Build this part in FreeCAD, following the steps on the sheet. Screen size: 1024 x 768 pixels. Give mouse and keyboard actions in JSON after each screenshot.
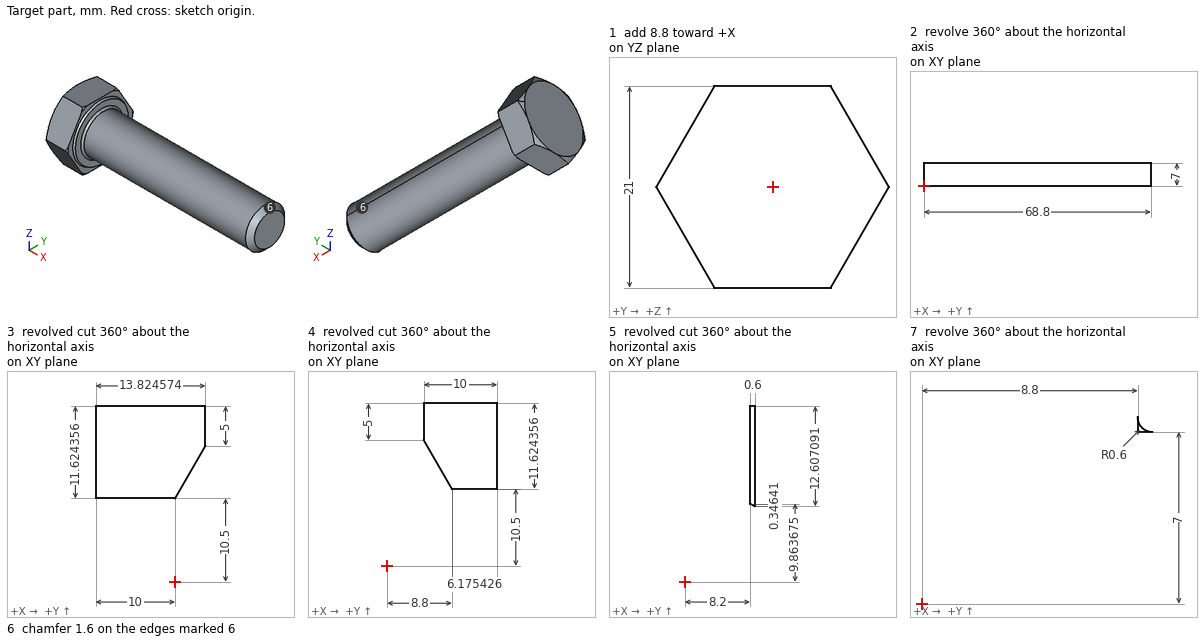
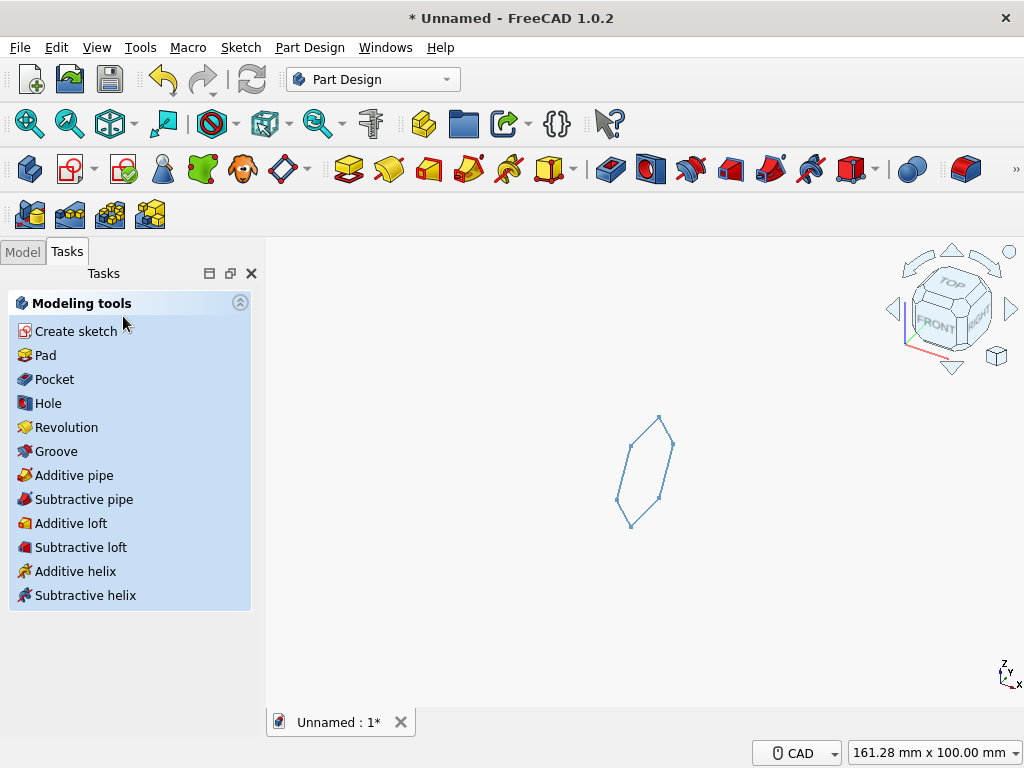
{"action": "left_click", "coordinate": [350, 170]}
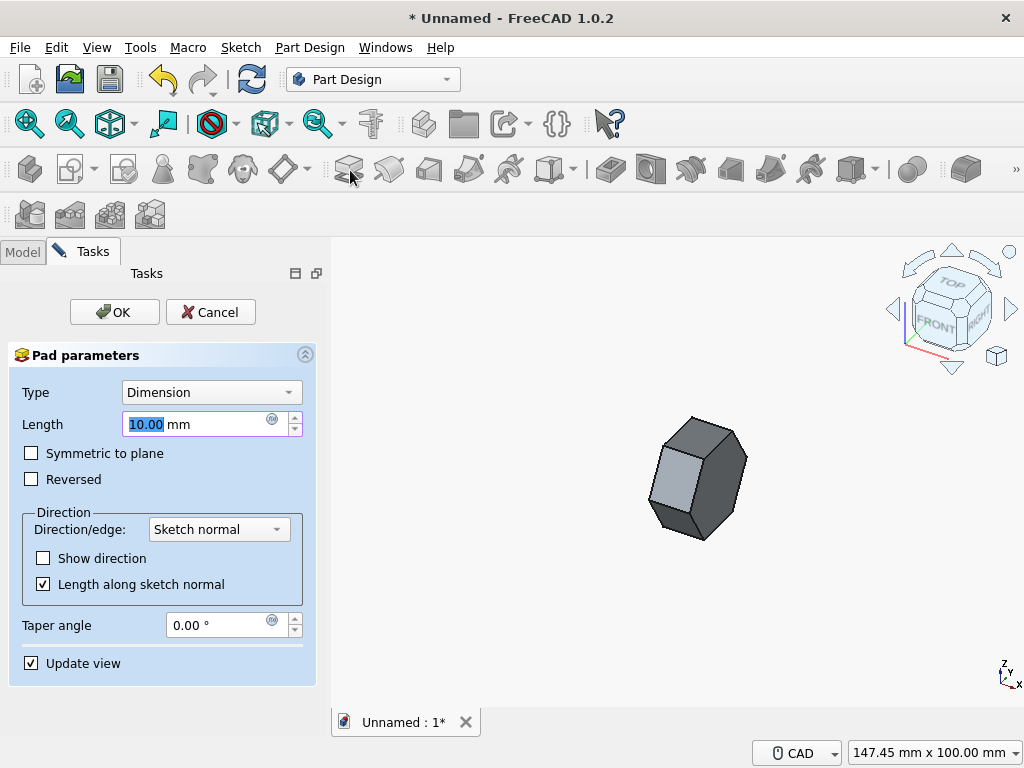
{"action": "type", "text": "8.8"}
{"action": "key", "text": "Tab"}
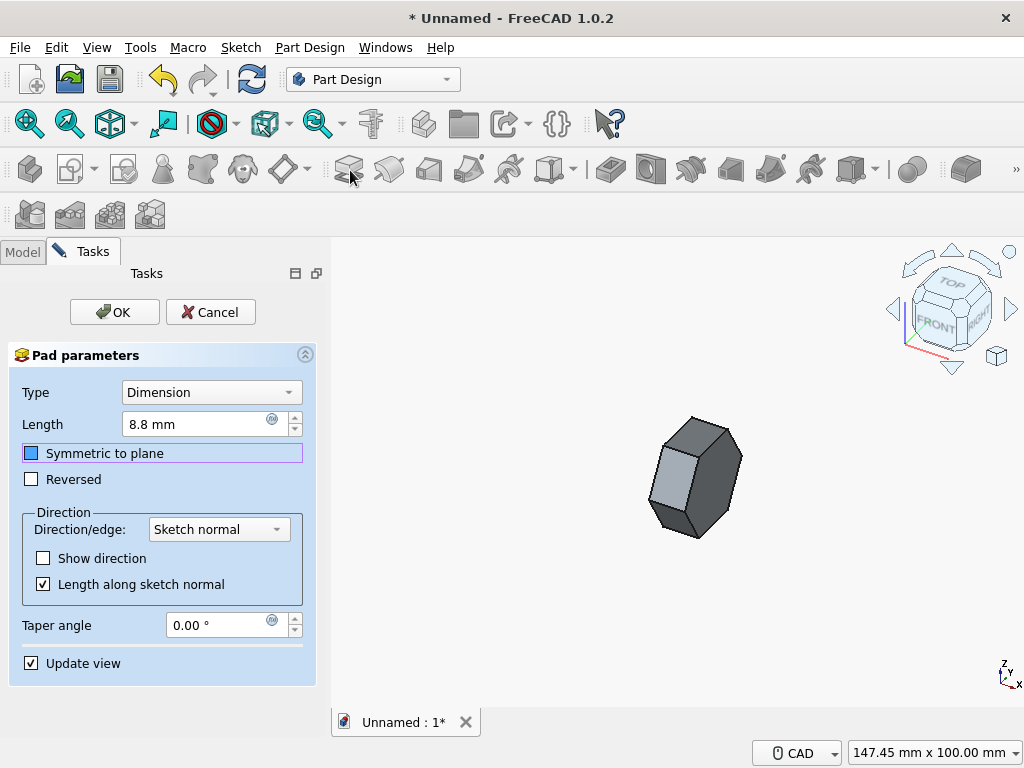
{"action": "left_click", "coordinate": [115, 312]}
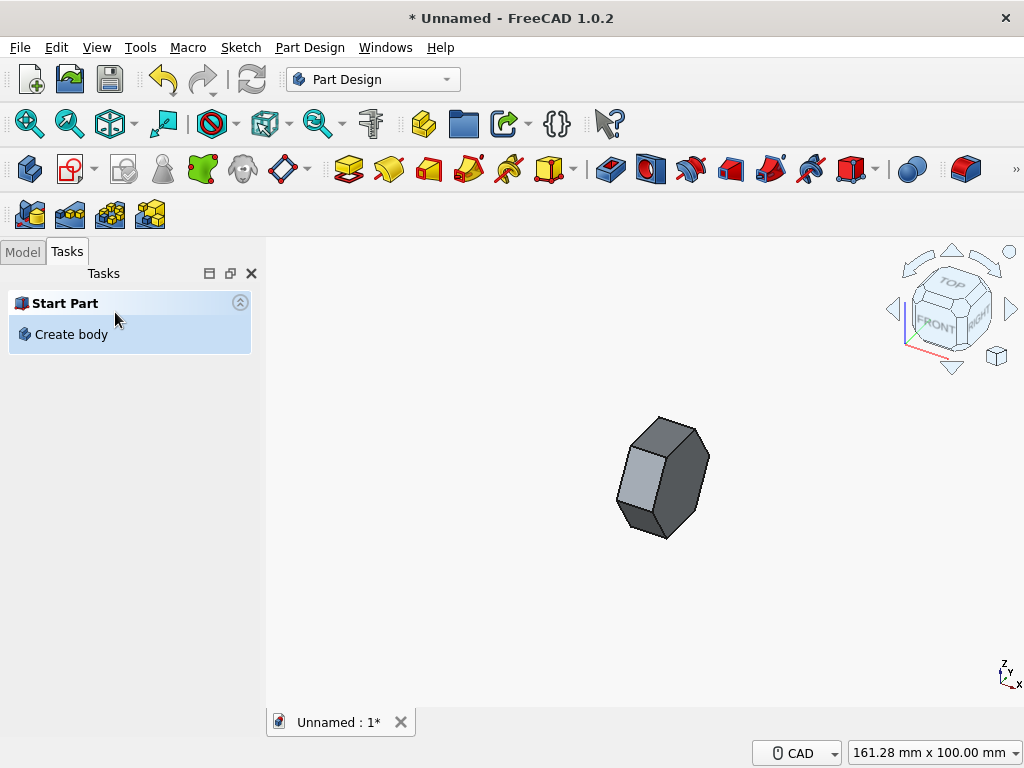
{"action": "left_click", "coordinate": [30, 124]}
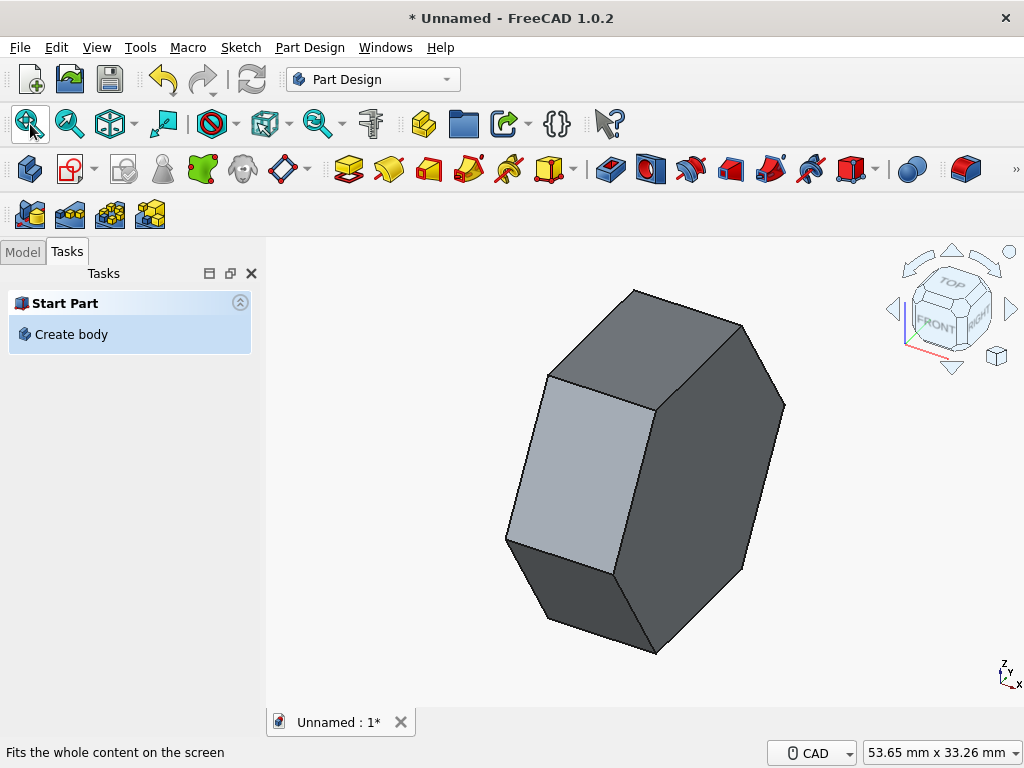
{"action": "left_click", "coordinate": [70, 170]}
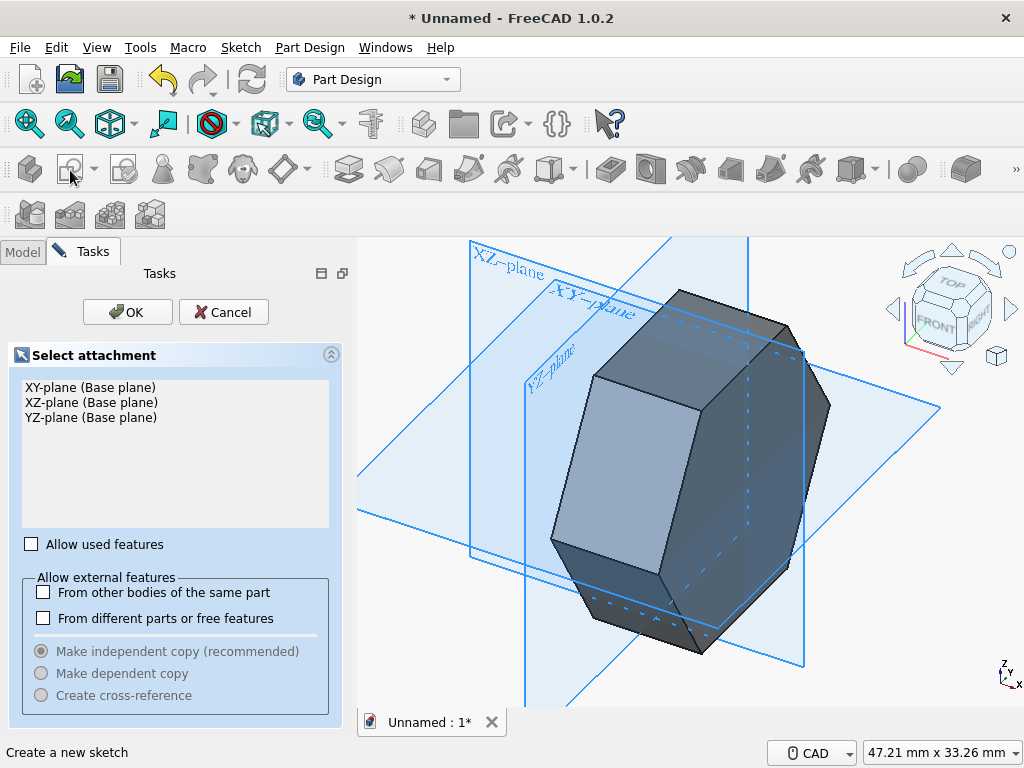
{"action": "left_click", "coordinate": [82, 388]}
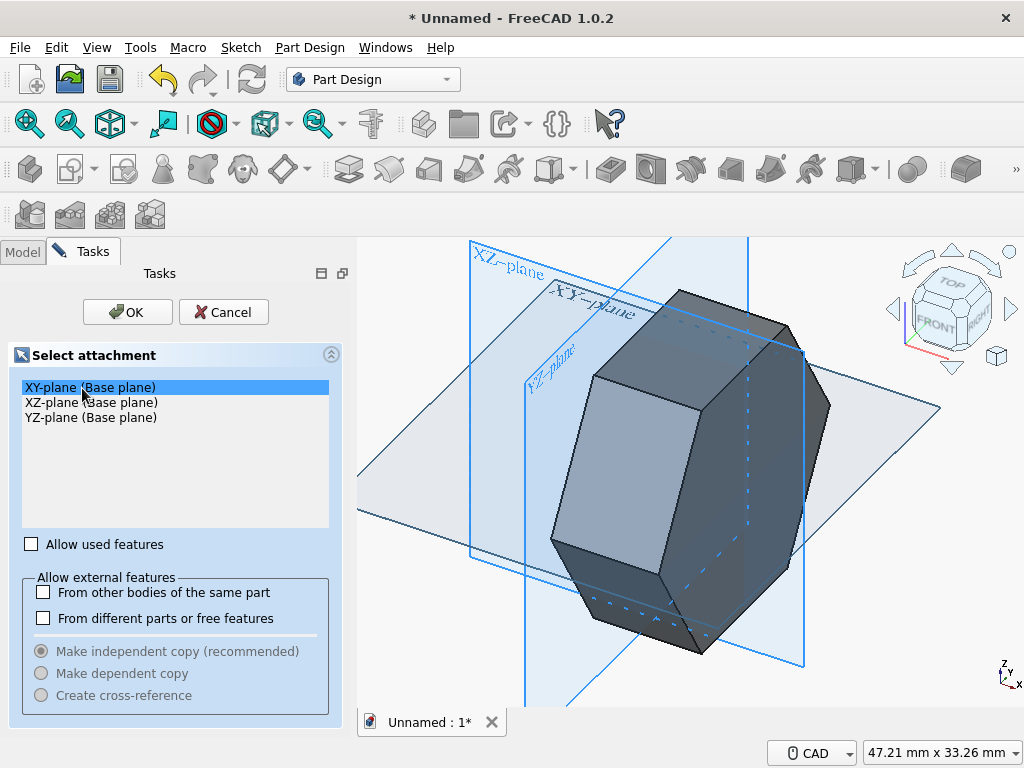
{"action": "left_click", "coordinate": [128, 312]}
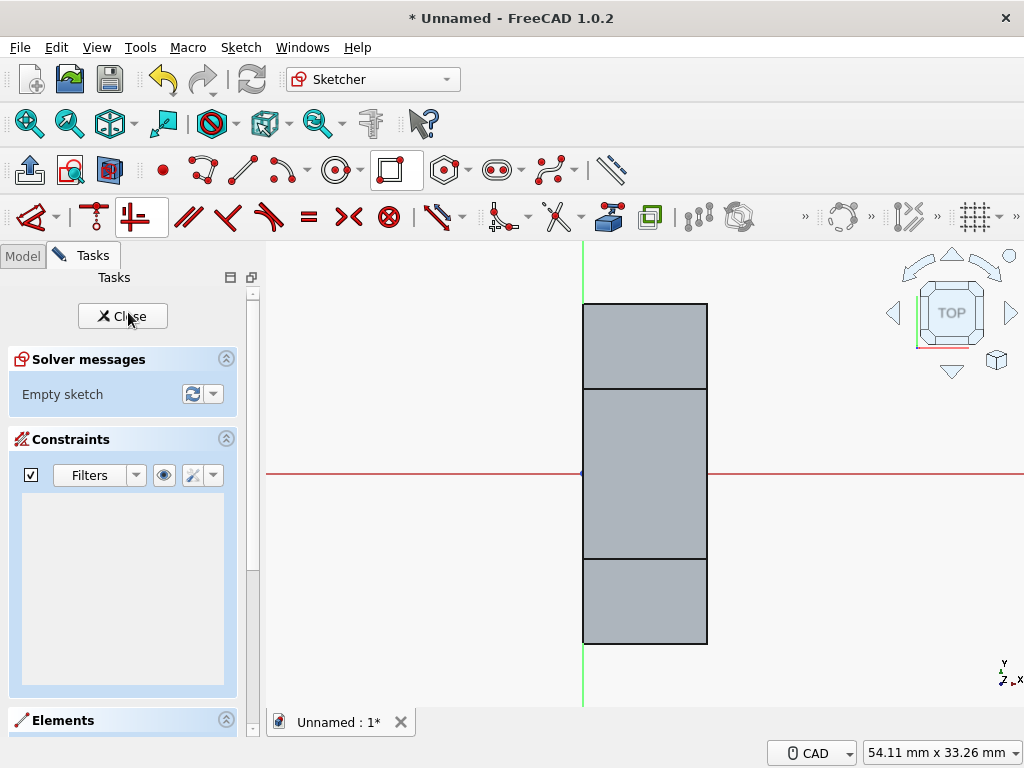
{"action": "key", "text": "q s"}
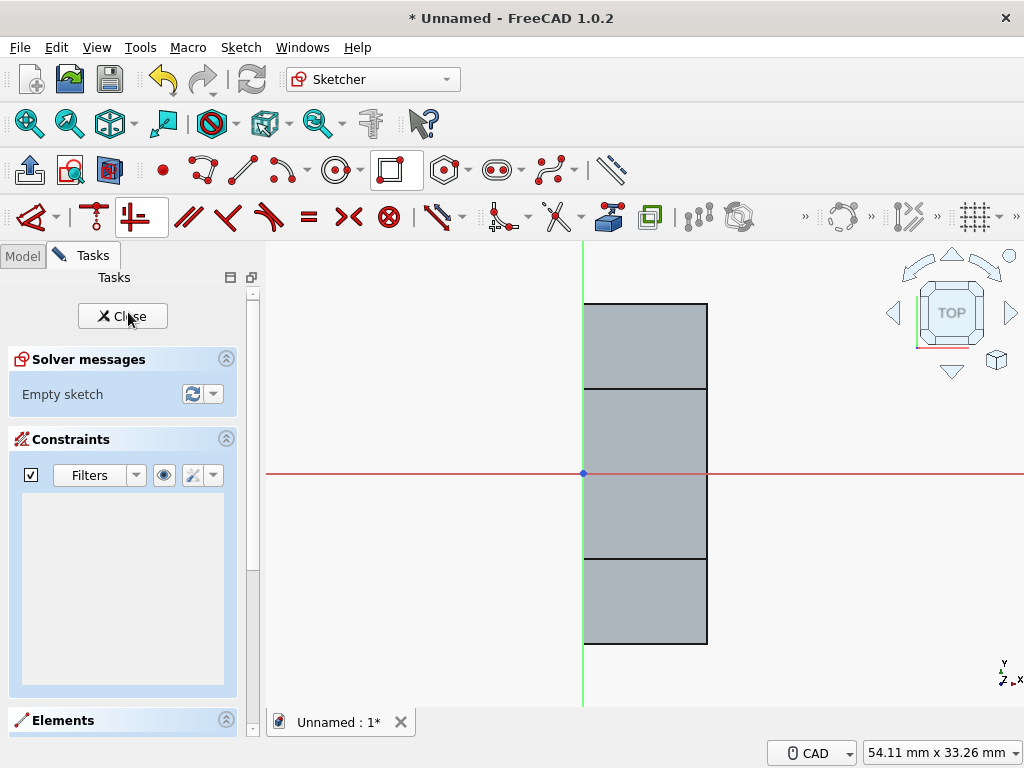
{"action": "scroll", "coordinate": [294, 503], "scroll_direction": "down", "scroll_amount": 5}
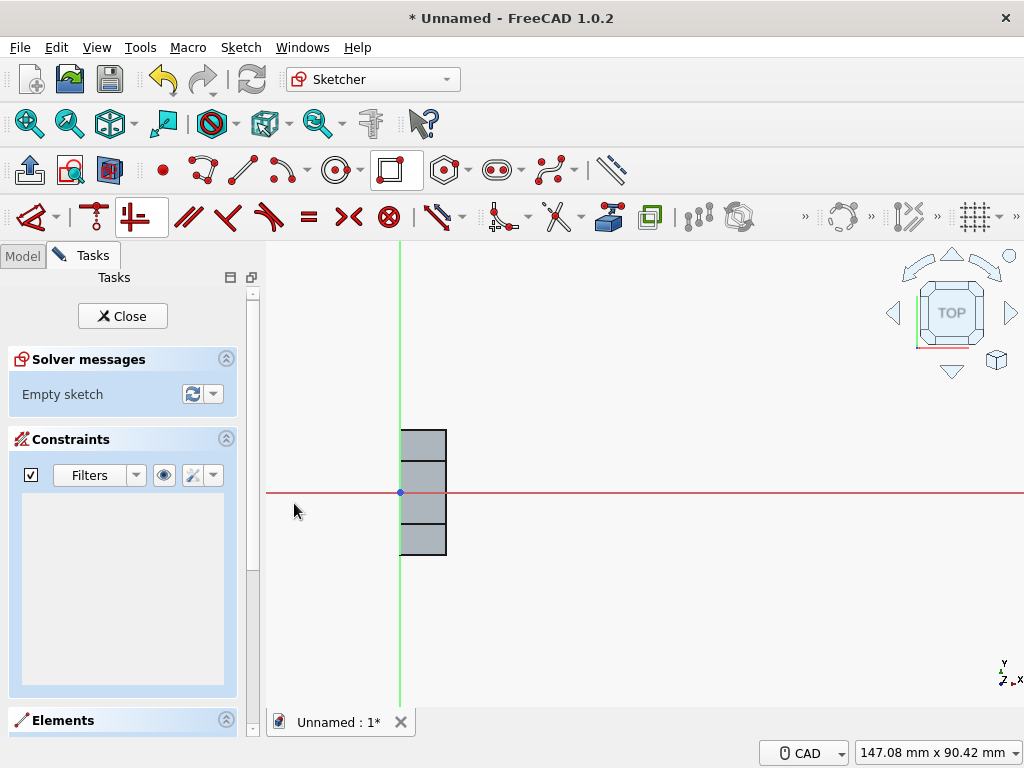
{"action": "left_click", "coordinate": [390, 170]}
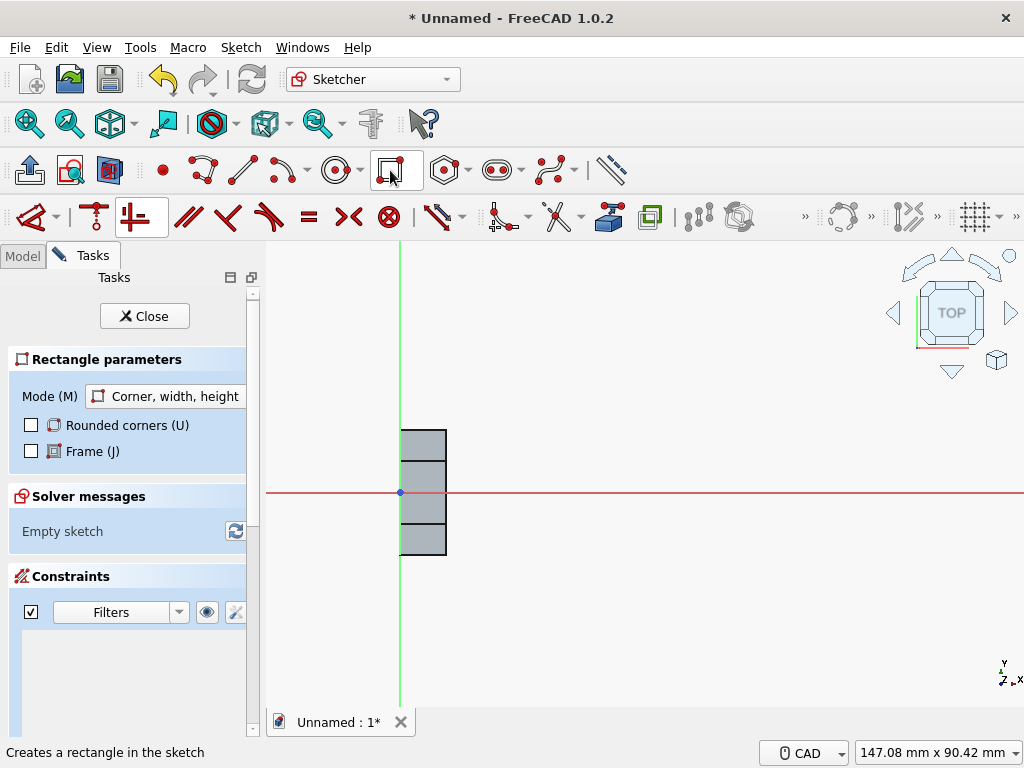
{"action": "left_click", "coordinate": [400, 493]}
{"action": "left_click", "coordinate": [755, 457]}
{"action": "key", "text": "Escape"}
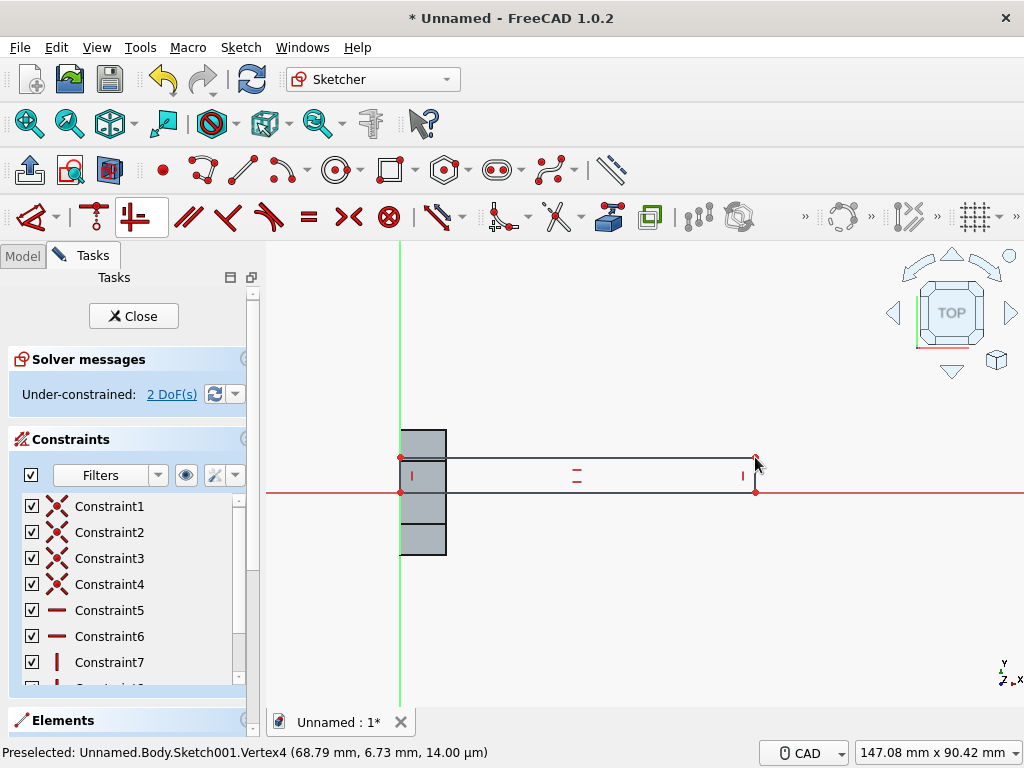
{"action": "scroll", "coordinate": [755, 482], "scroll_direction": "up", "scroll_amount": 2}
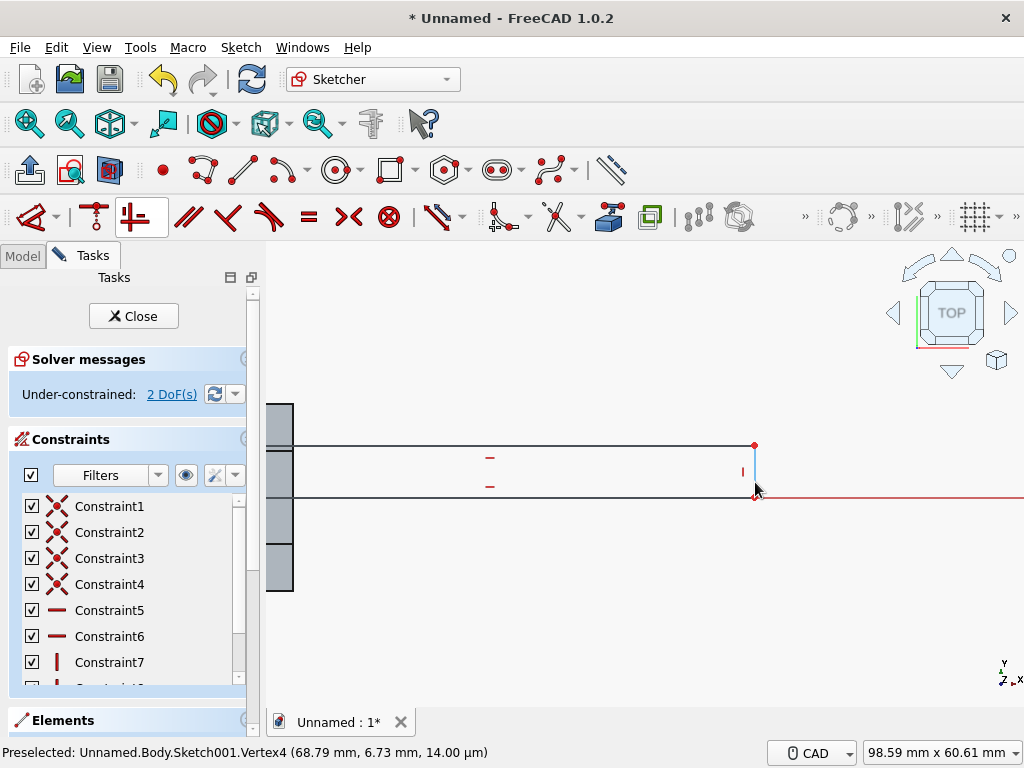
{"action": "left_click", "coordinate": [755, 482]}